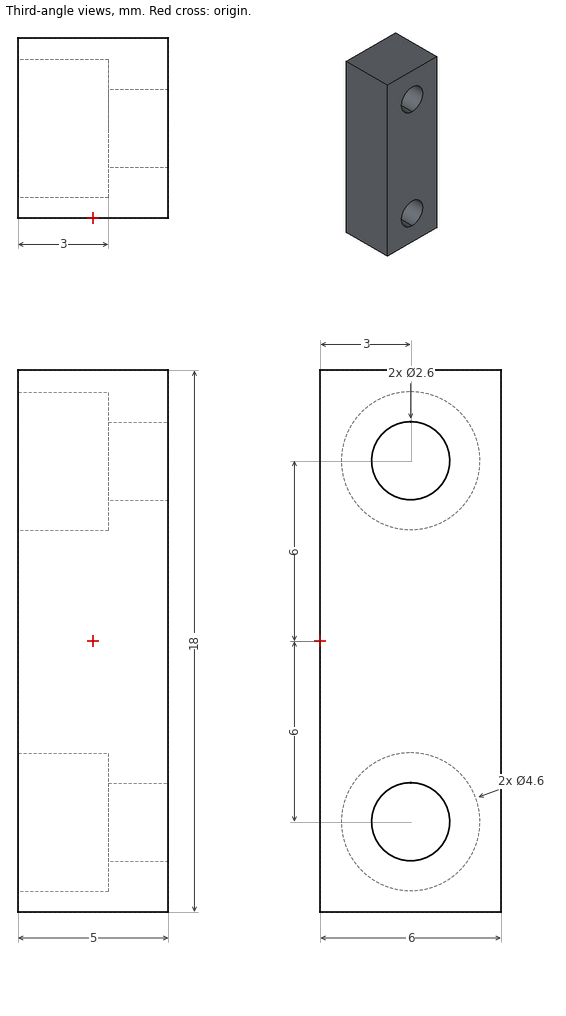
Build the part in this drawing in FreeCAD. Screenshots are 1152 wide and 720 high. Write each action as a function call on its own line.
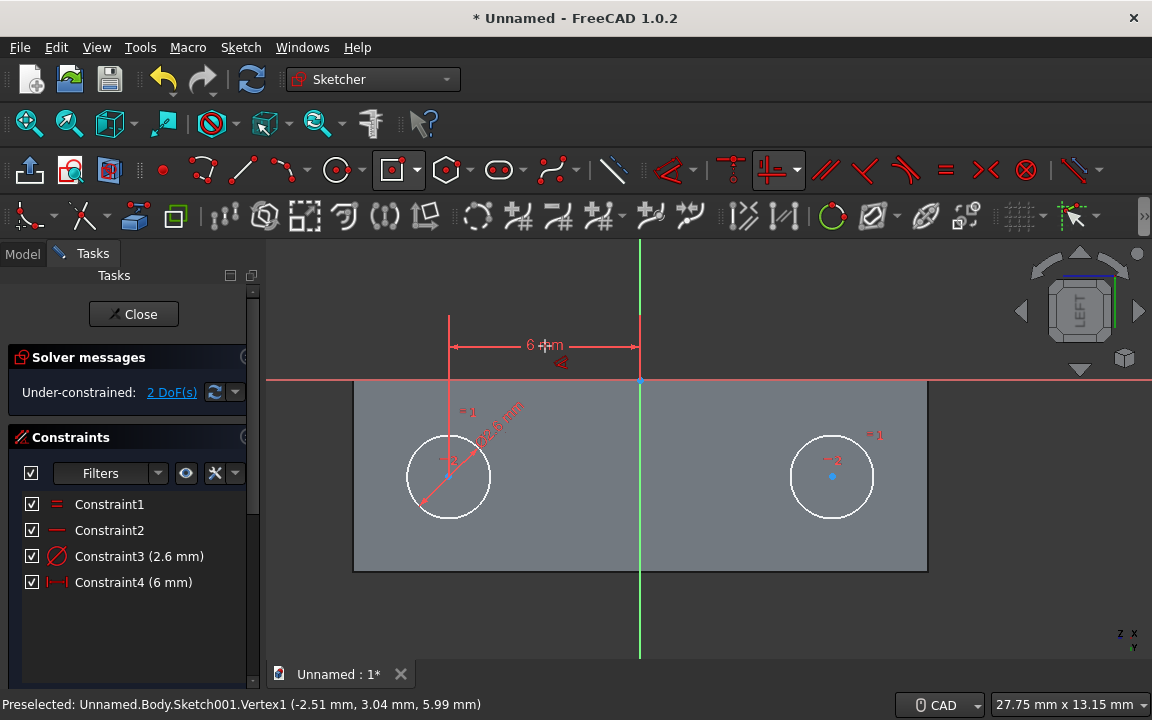
click(449, 477)
click(415, 429)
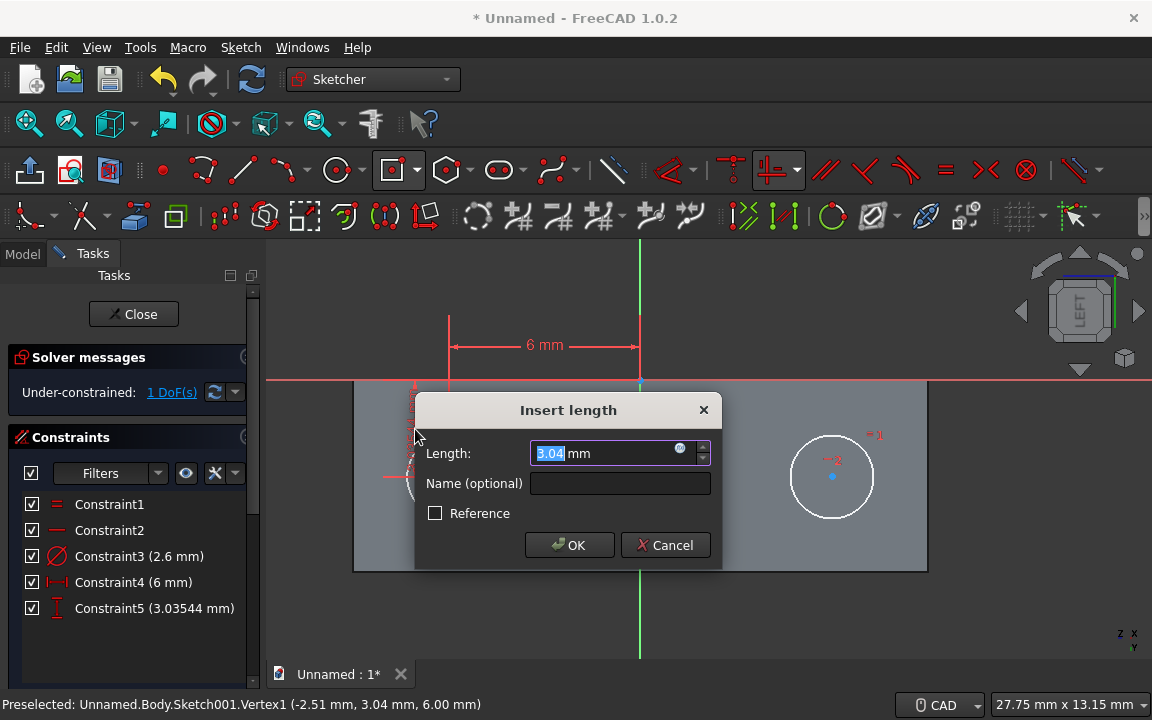
text(3)
key(Return)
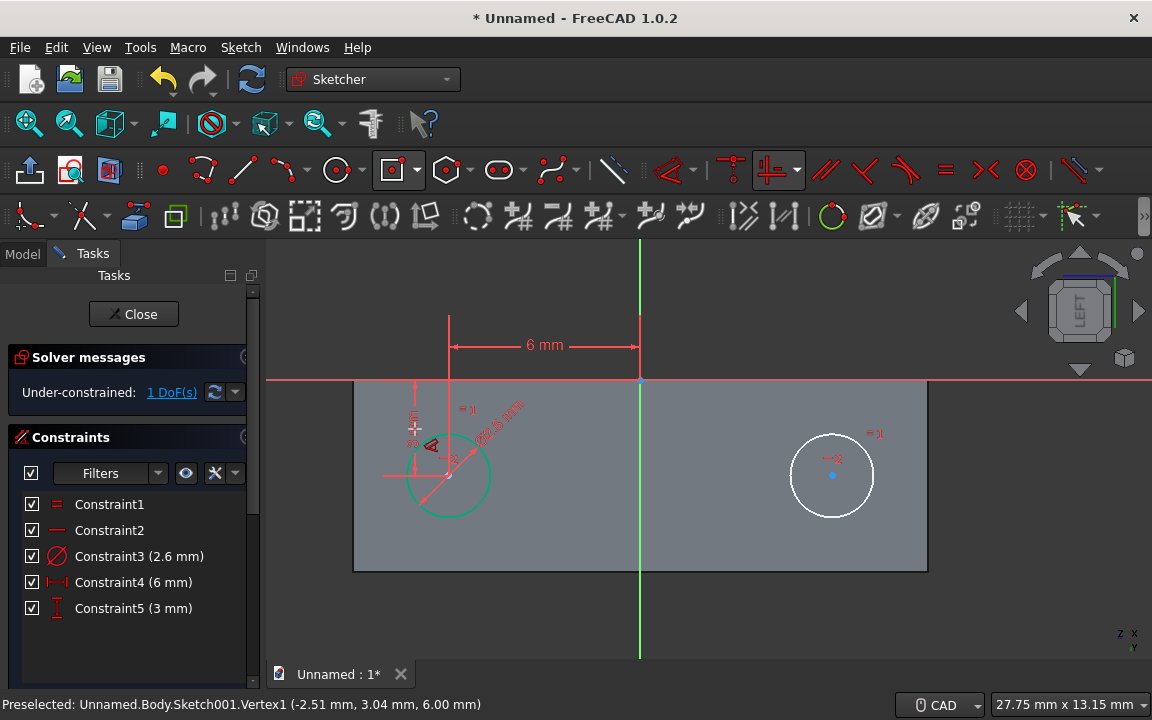
click(832, 476)
click(736, 346)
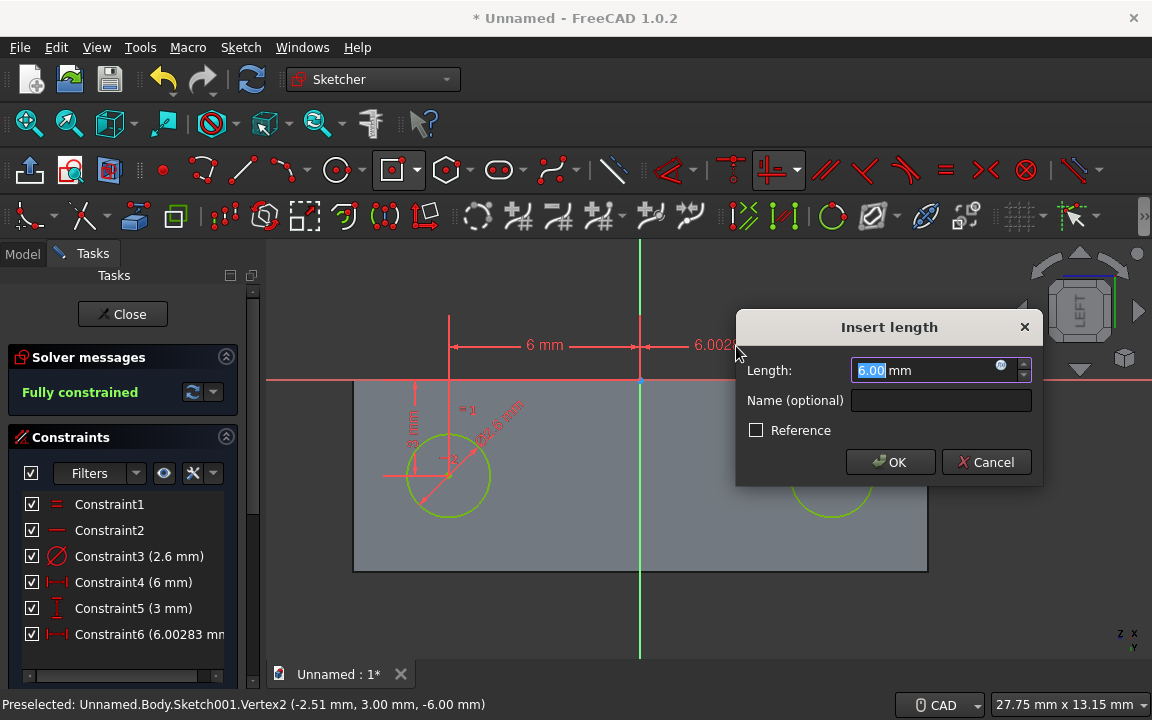
text(6)
key(Return)
key(Escape)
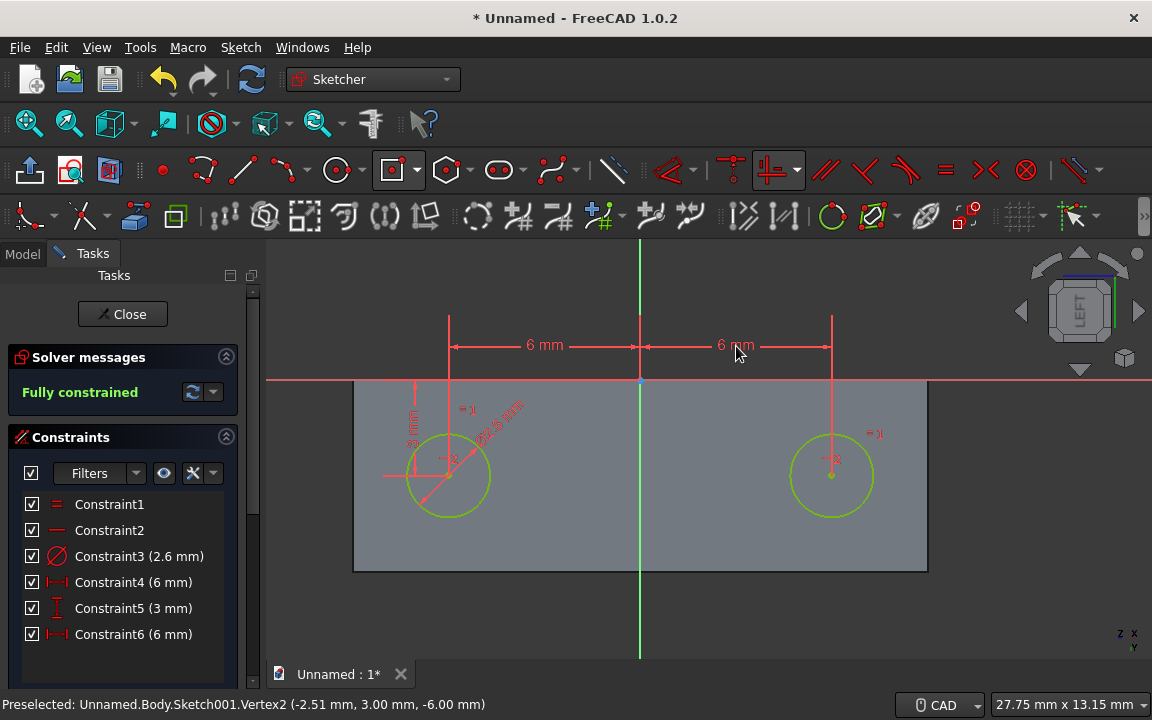
click(123, 314)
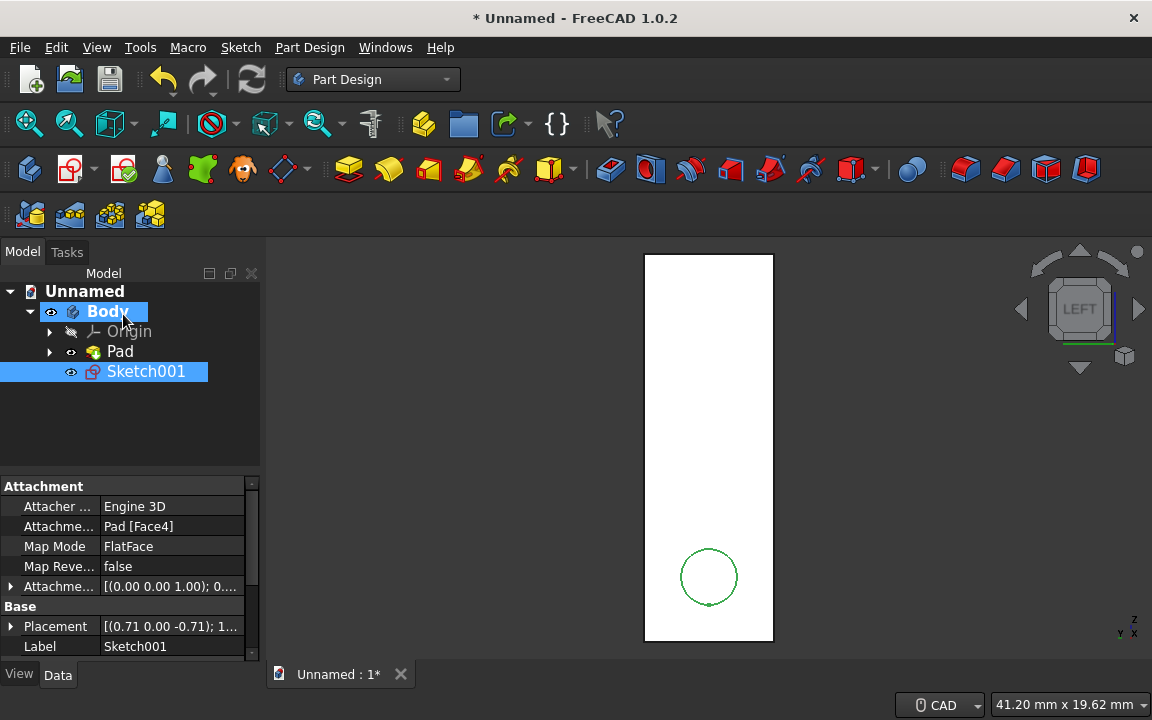
click(612, 170)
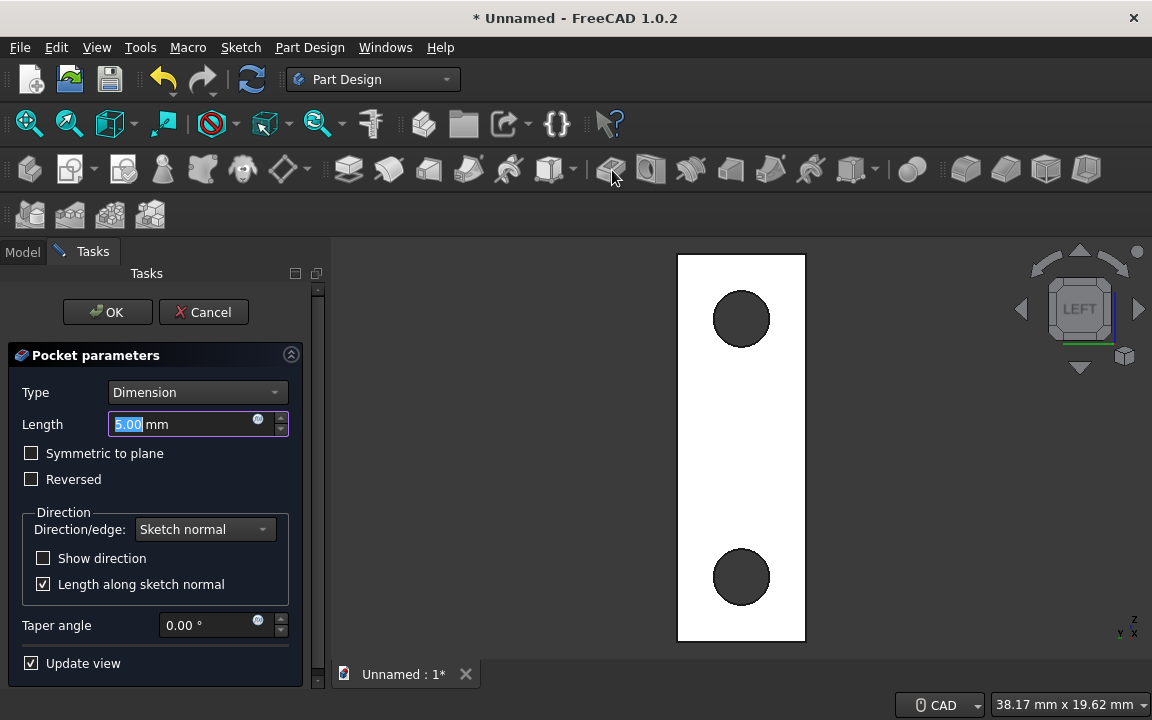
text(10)
key(Tab)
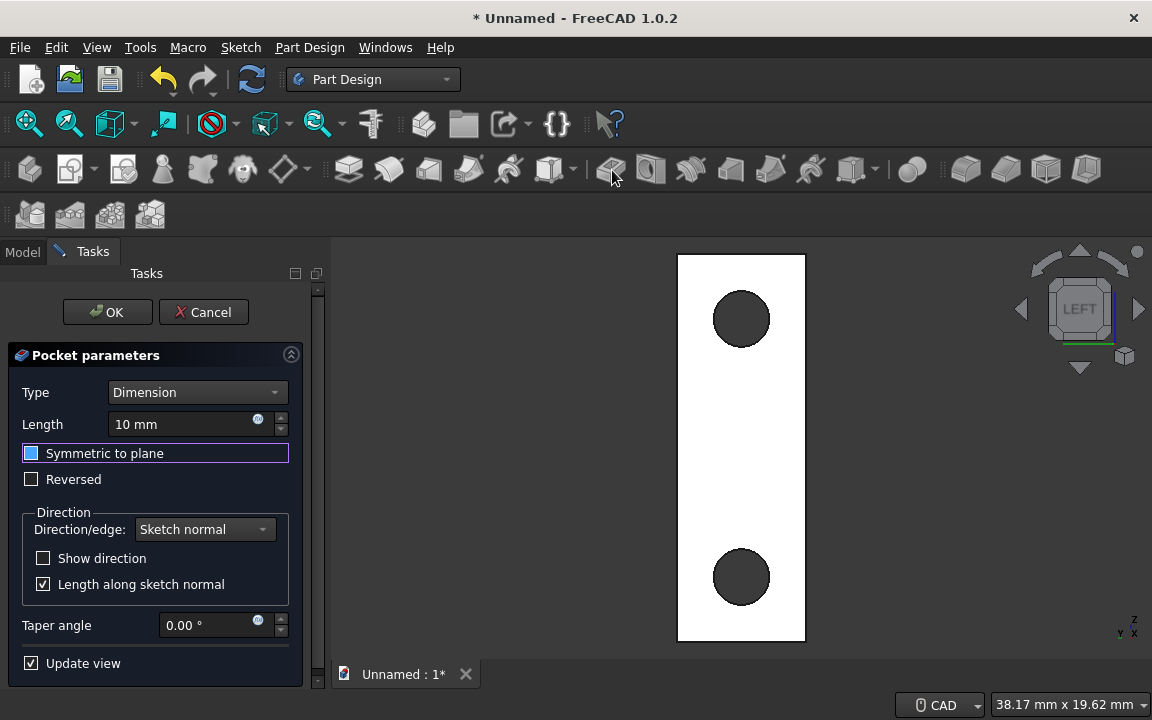
click(108, 312)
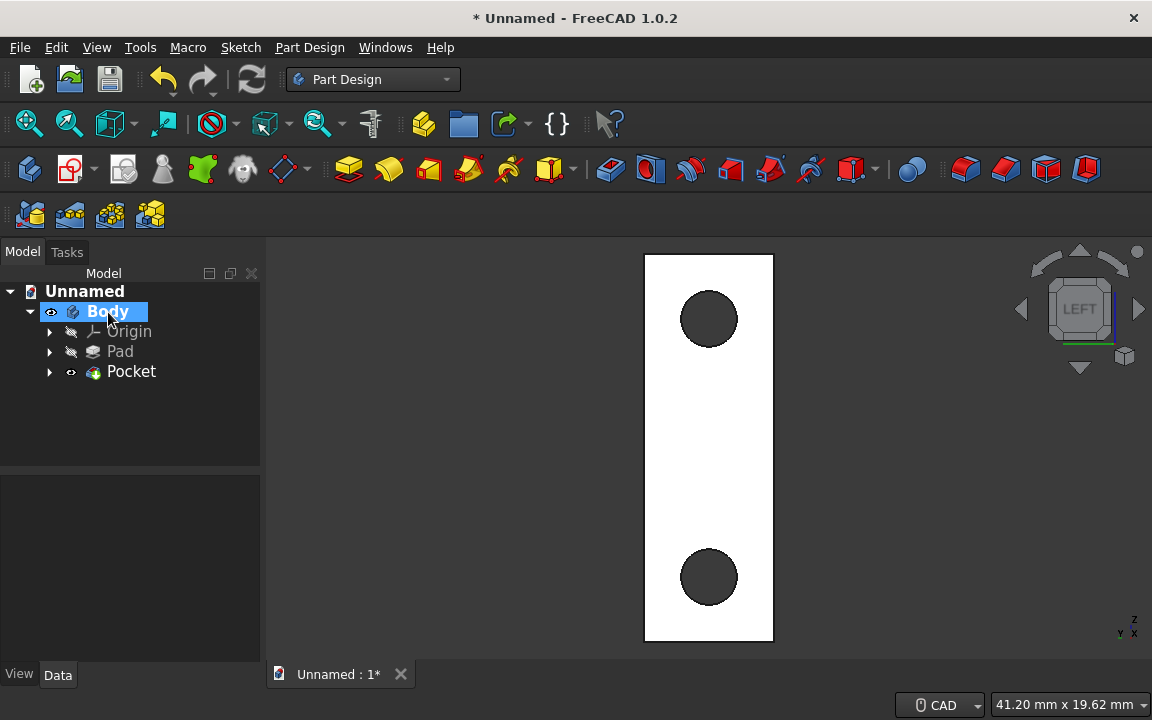
click(709, 447)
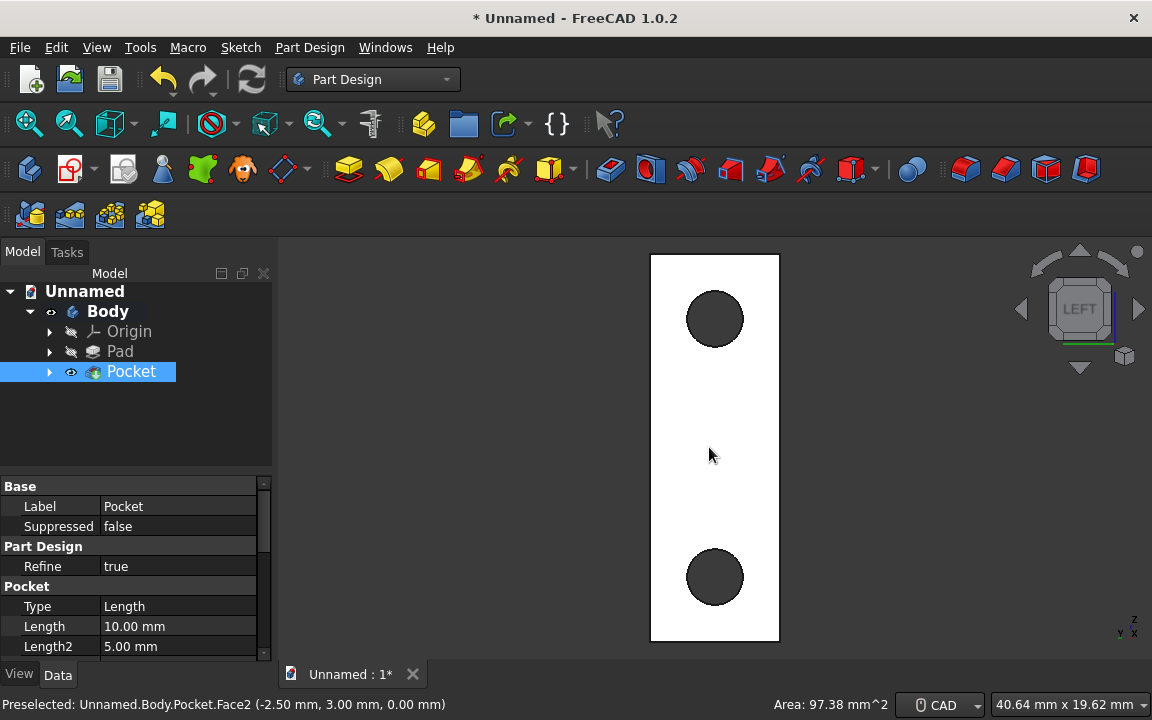
click(70, 170)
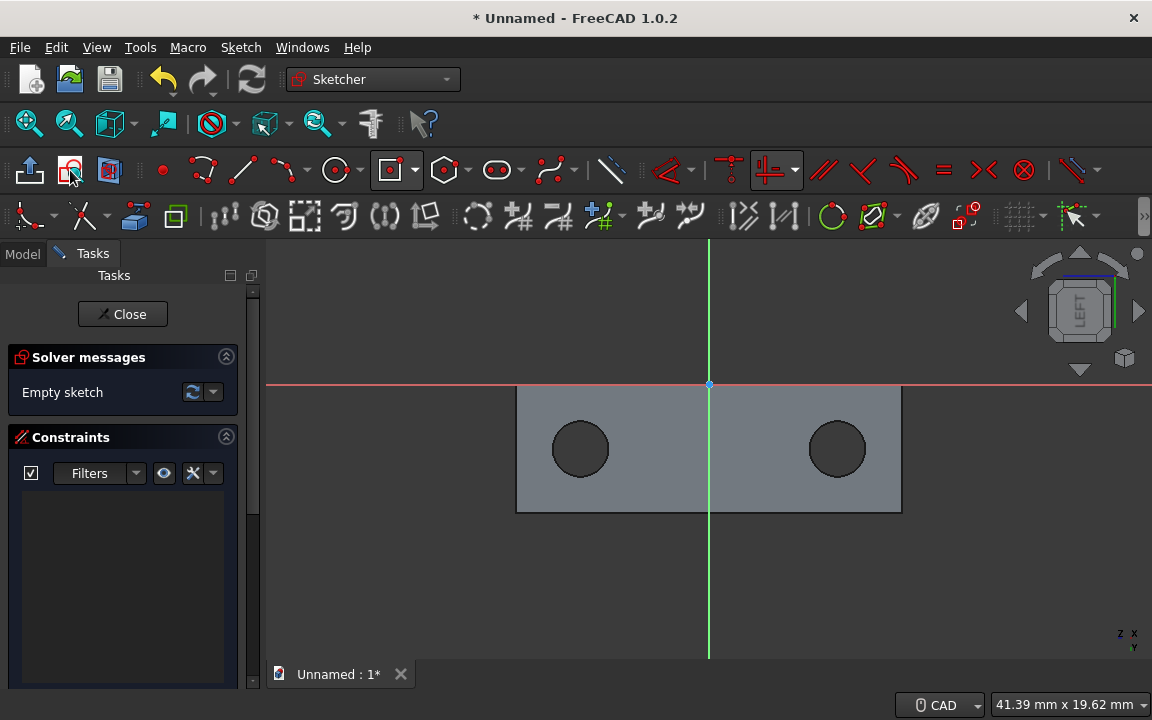
scroll(848, 426, up, 2)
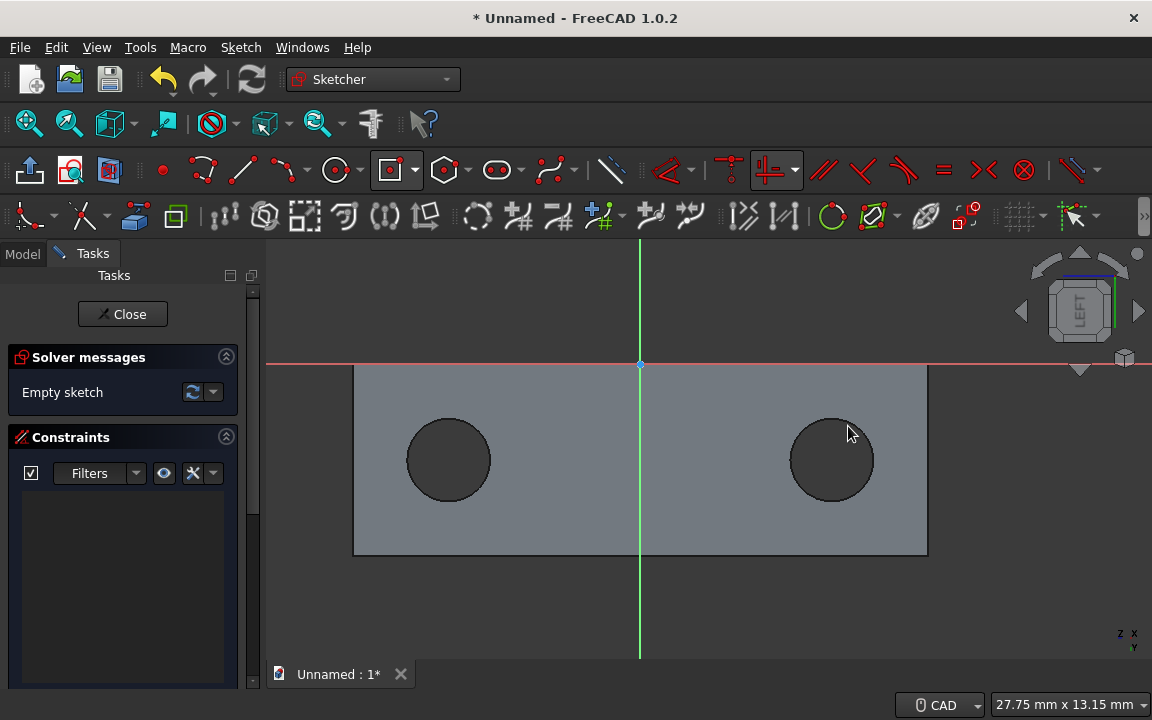
click(336, 170)